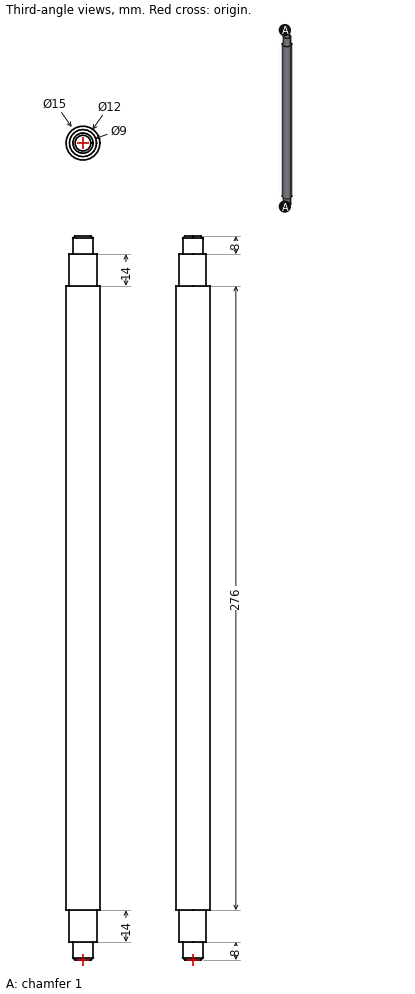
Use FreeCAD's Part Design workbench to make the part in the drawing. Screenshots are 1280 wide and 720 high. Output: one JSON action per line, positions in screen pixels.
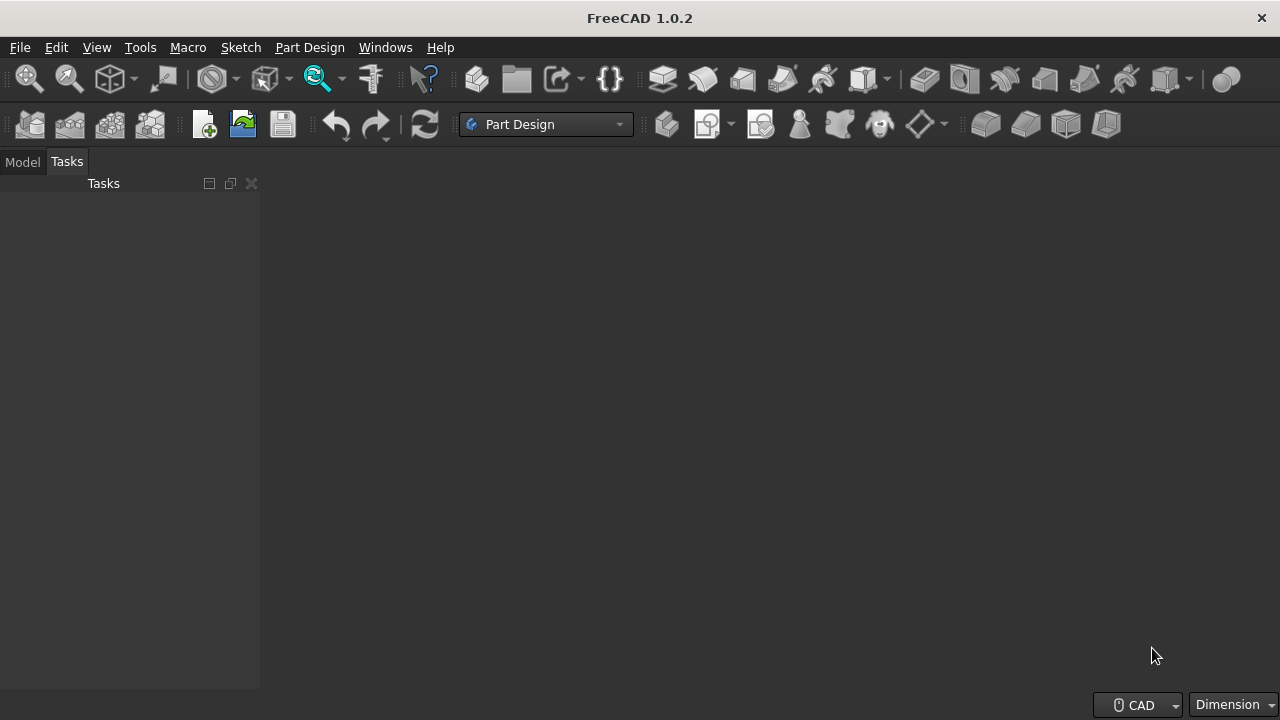
{"action": "key", "text": "ctrl+n"}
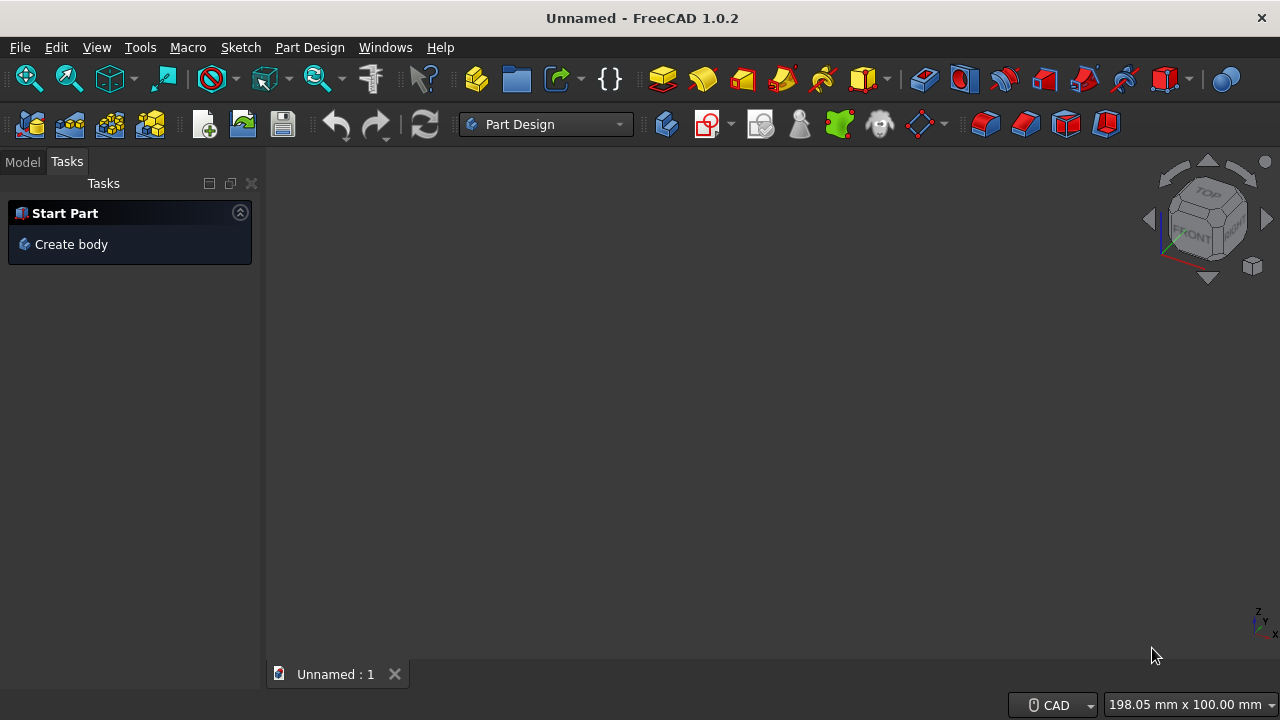
{"action": "left_click", "coordinate": [708, 124]}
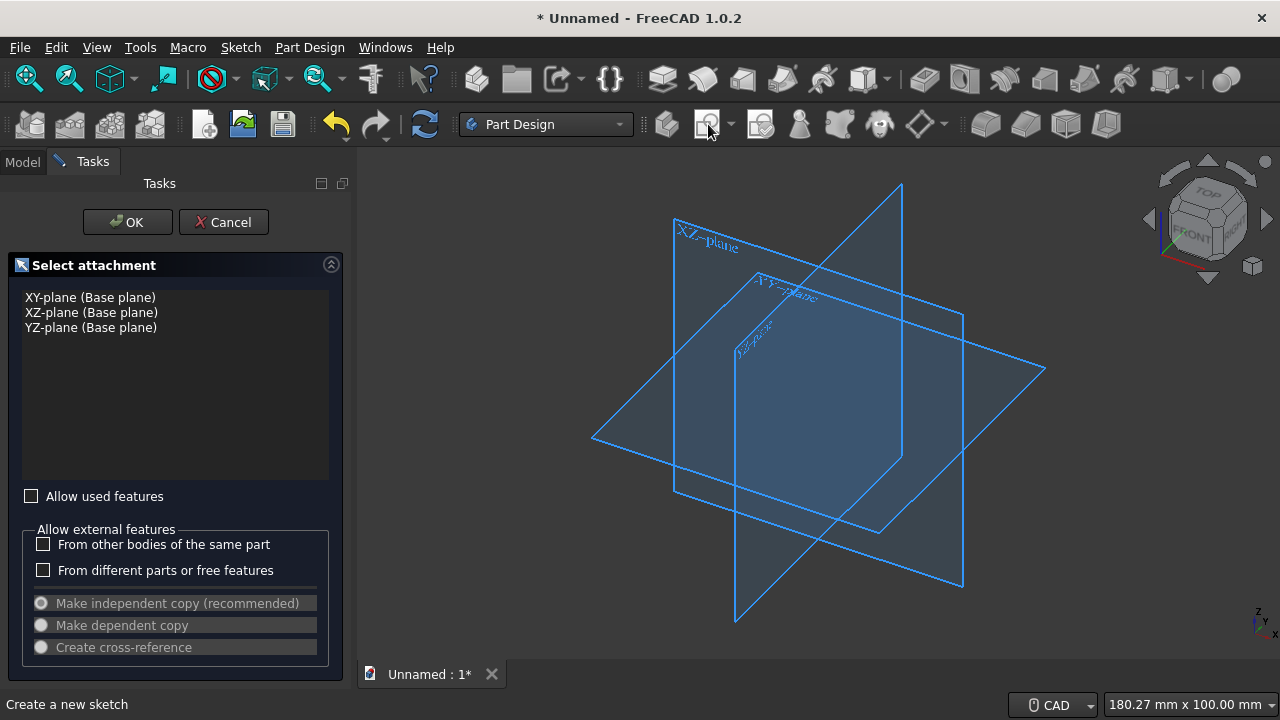
{"action": "left_click", "coordinate": [82, 298]}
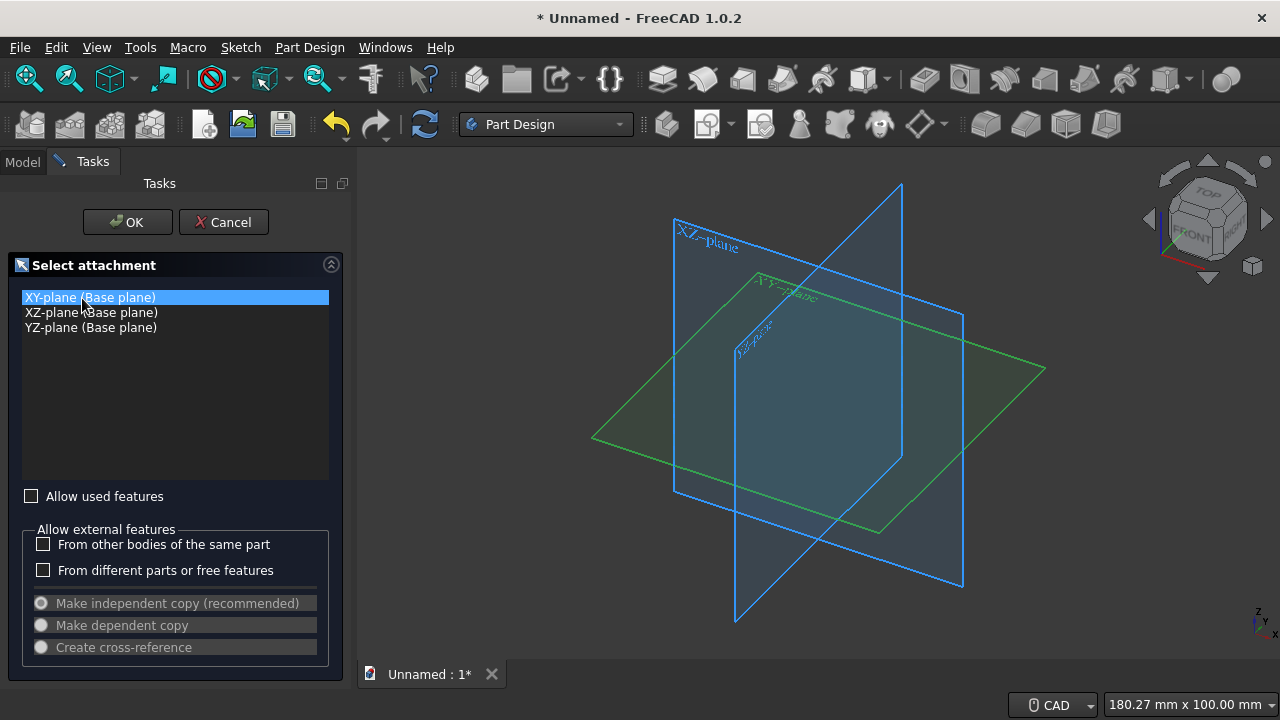
{"action": "left_click", "coordinate": [128, 222]}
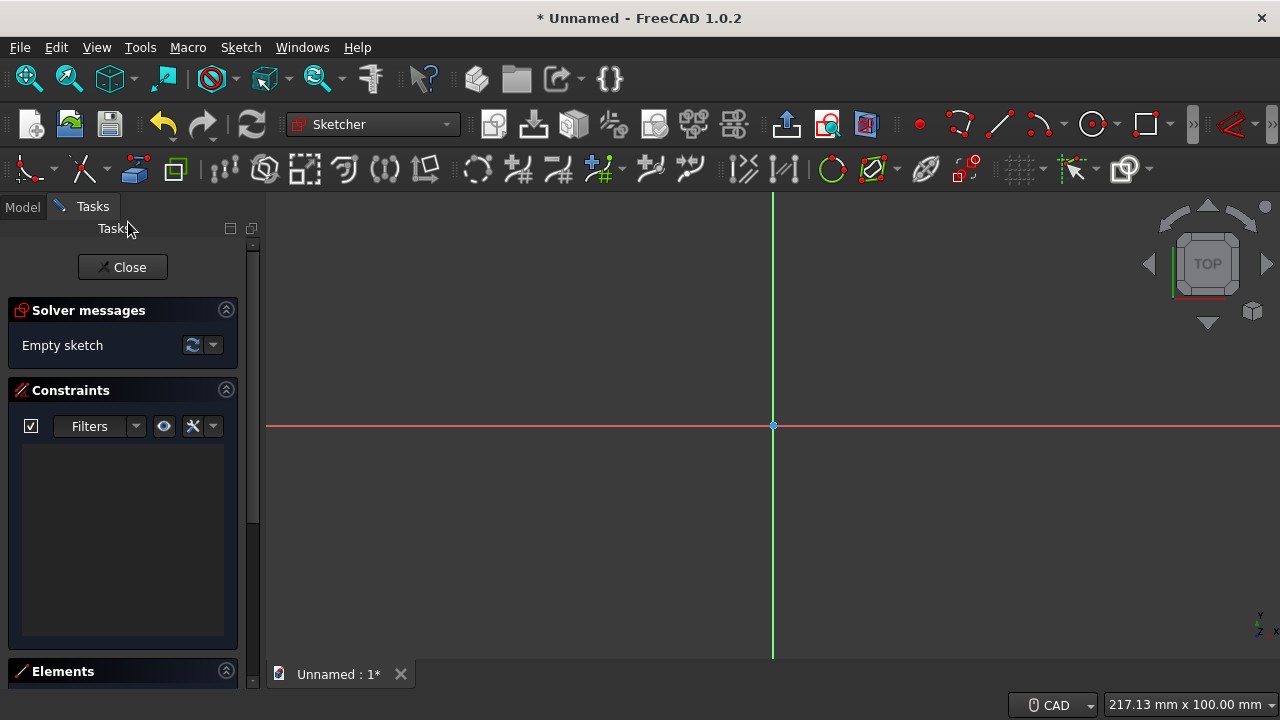
{"action": "scroll", "coordinate": [784, 426], "scroll_direction": "up", "scroll_amount": 10}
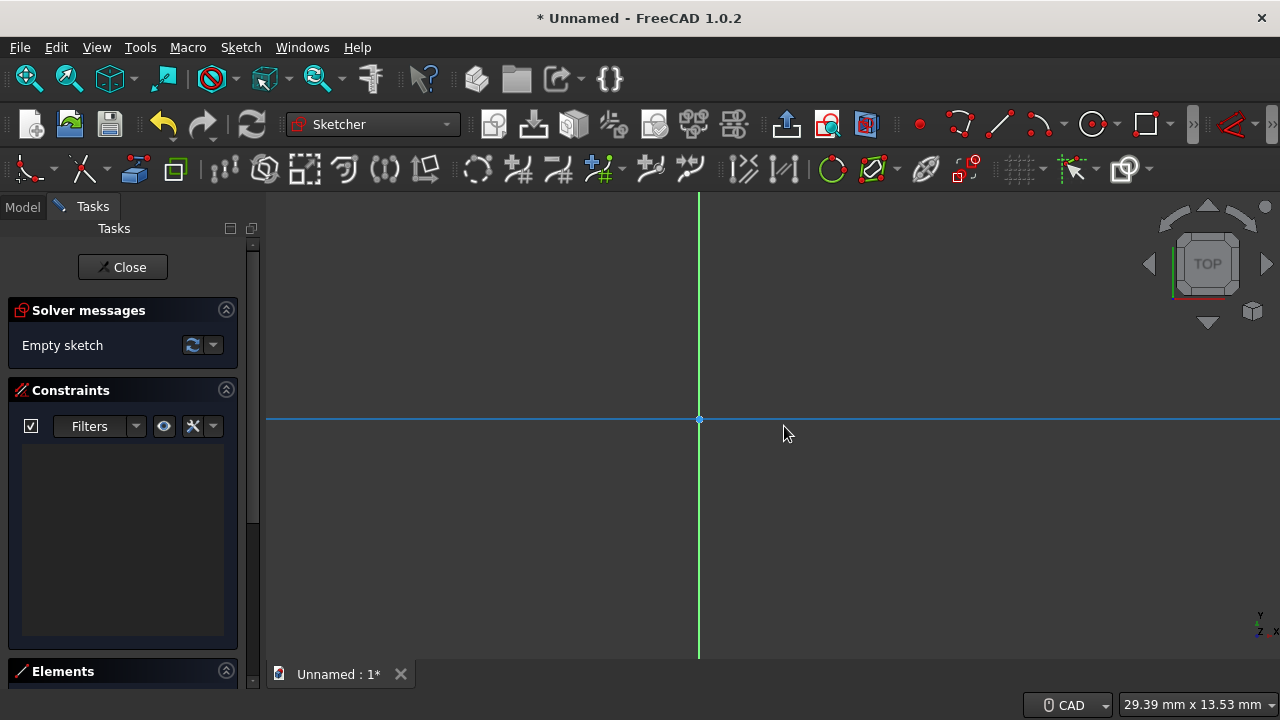
{"action": "left_click", "coordinate": [1094, 124]}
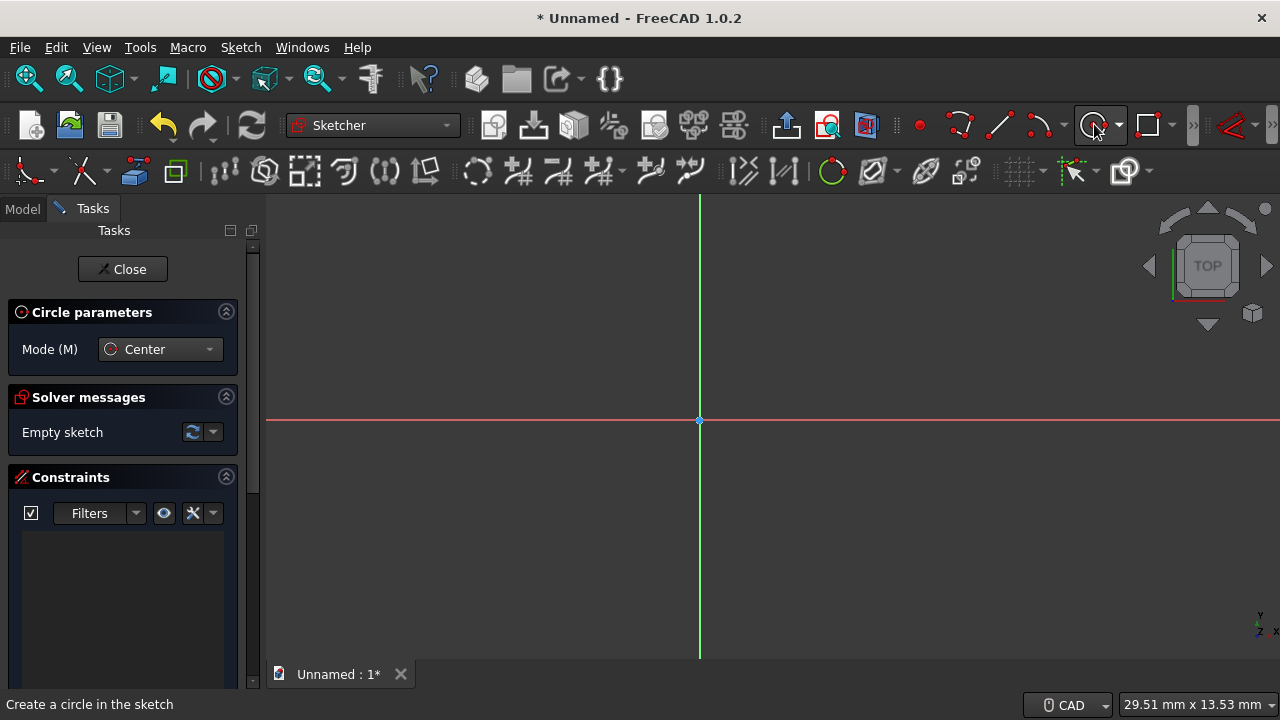
{"action": "left_click", "coordinate": [700, 420]}
{"action": "left_click", "coordinate": [809, 311]}
{"action": "key", "text": "Escape"}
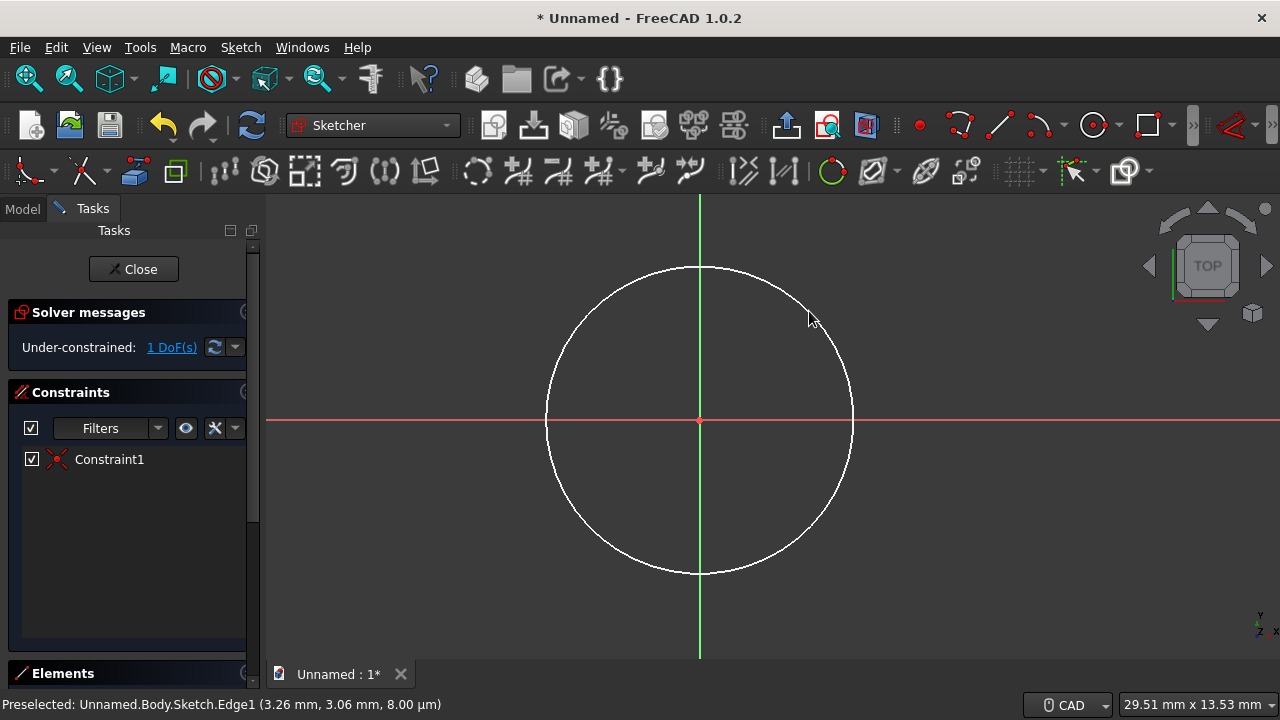
{"action": "key", "text": "d"}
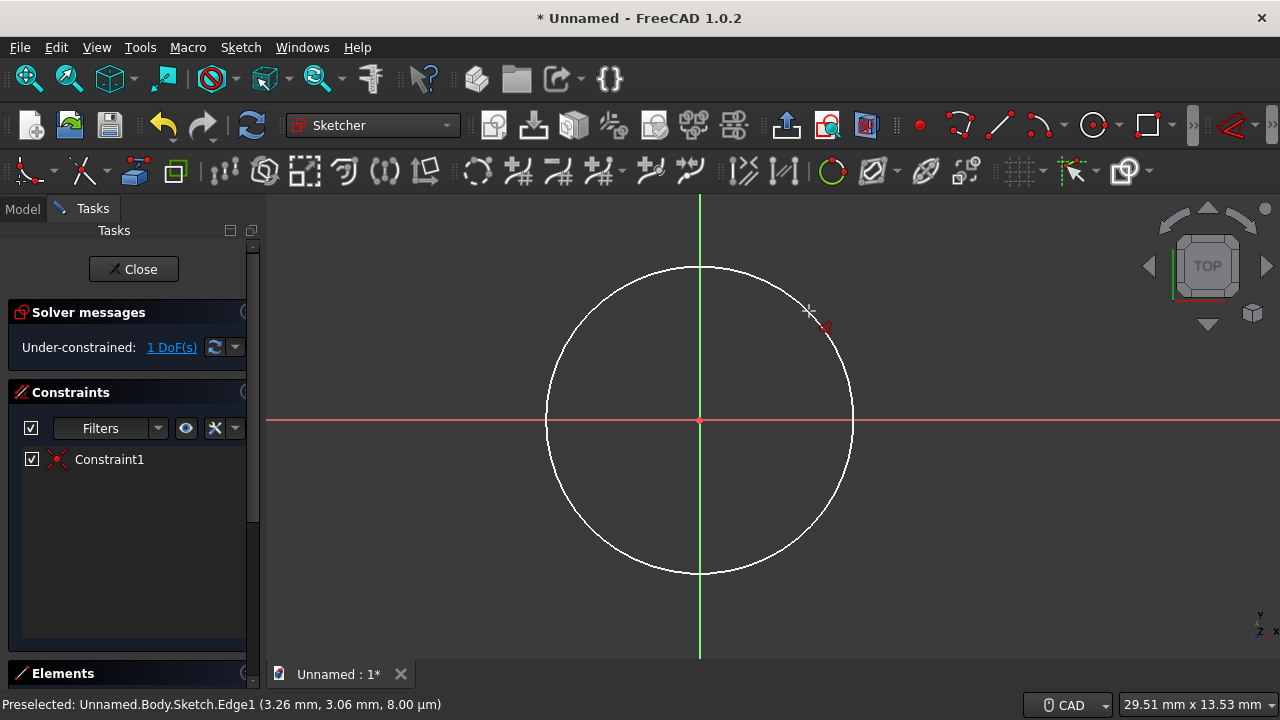
{"action": "left_click", "coordinate": [808, 311]}
{"action": "left_click", "coordinate": [831, 288]}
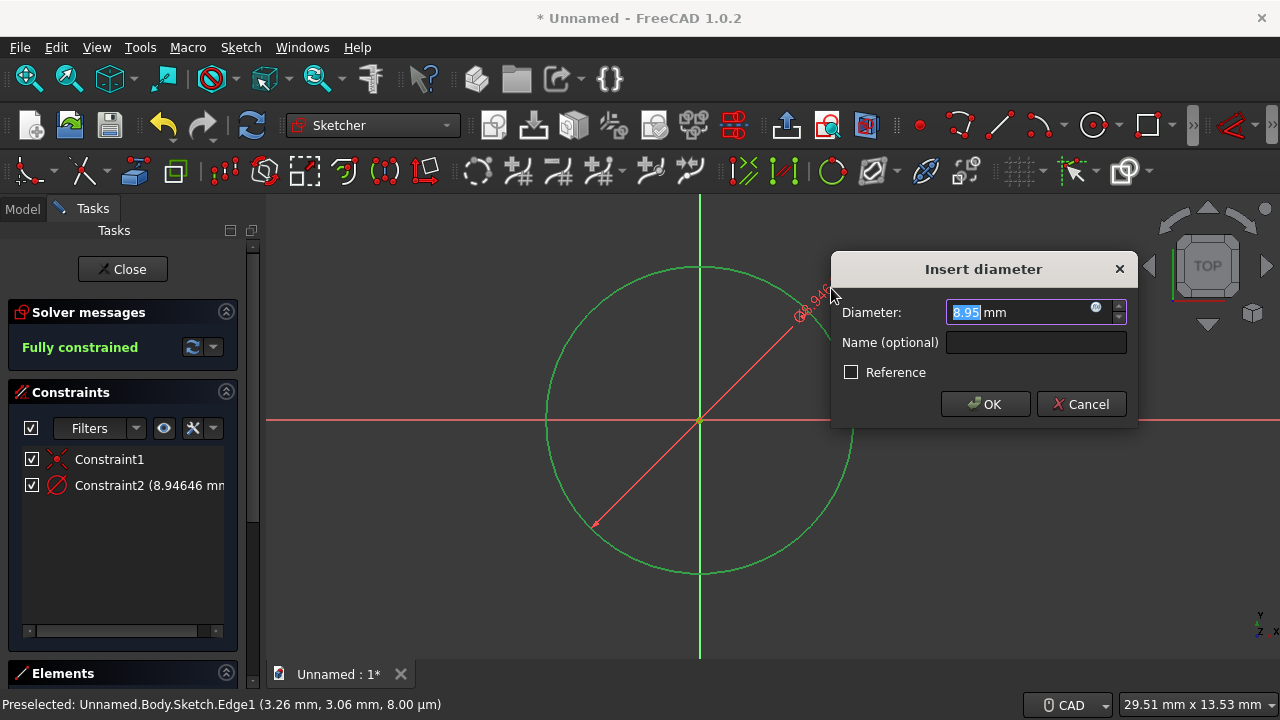
{"action": "type", "text": "9"}
{"action": "key", "text": "Return"}
{"action": "key", "text": "Escape"}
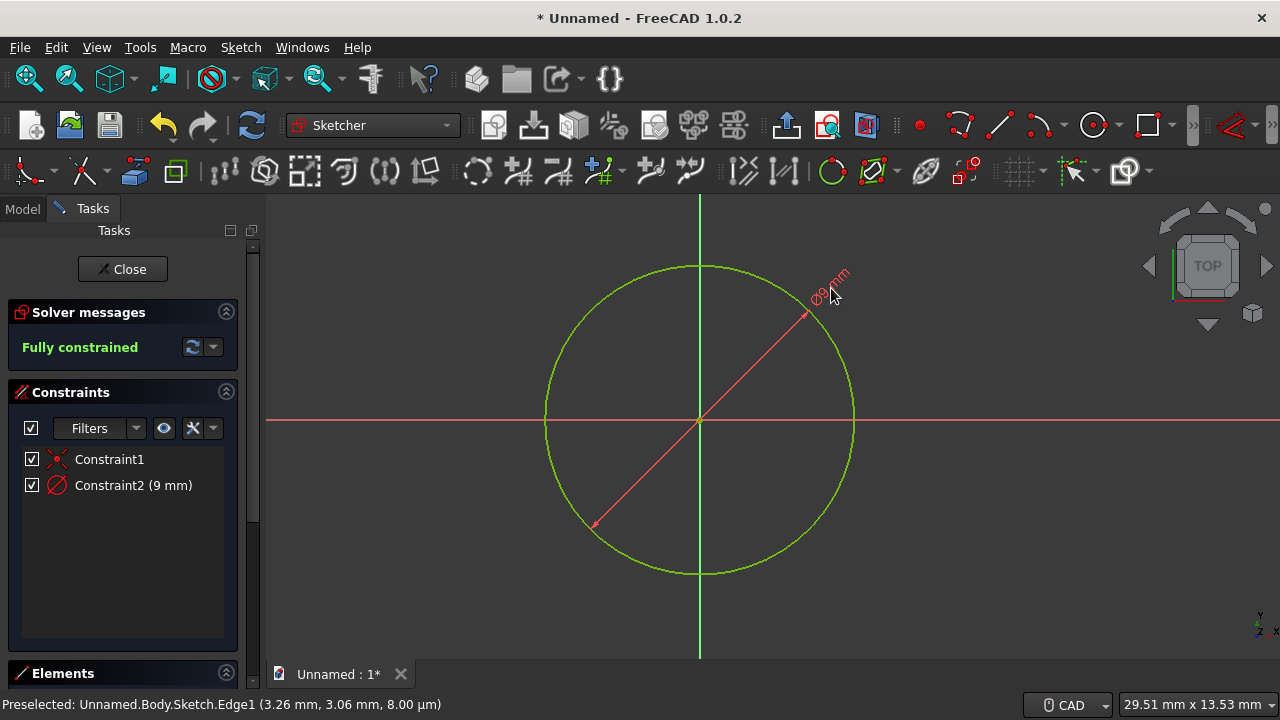
{"action": "left_click", "coordinate": [123, 269]}